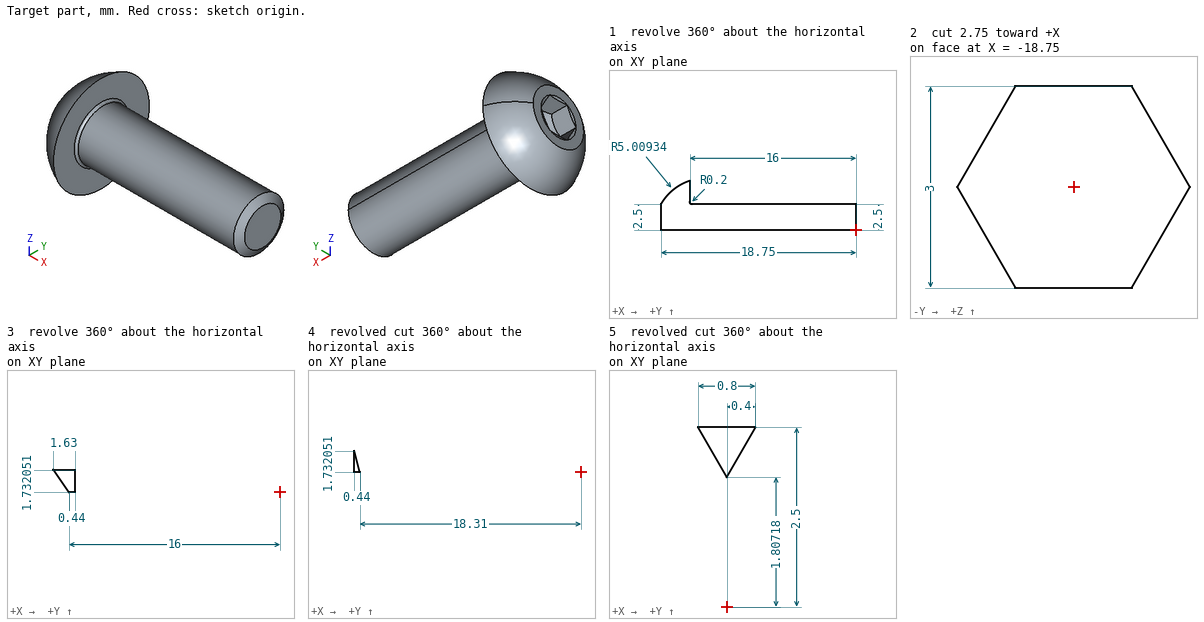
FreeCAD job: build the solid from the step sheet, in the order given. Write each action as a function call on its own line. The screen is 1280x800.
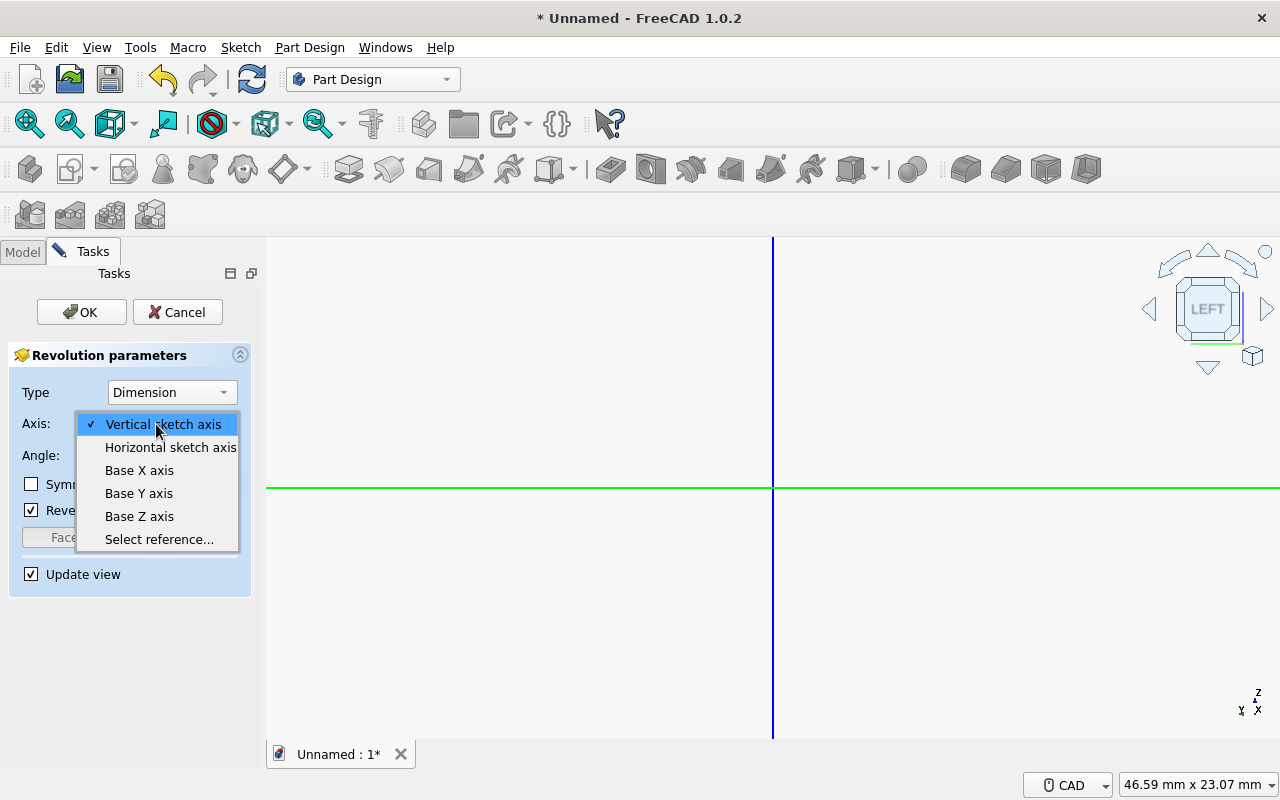
click(156, 448)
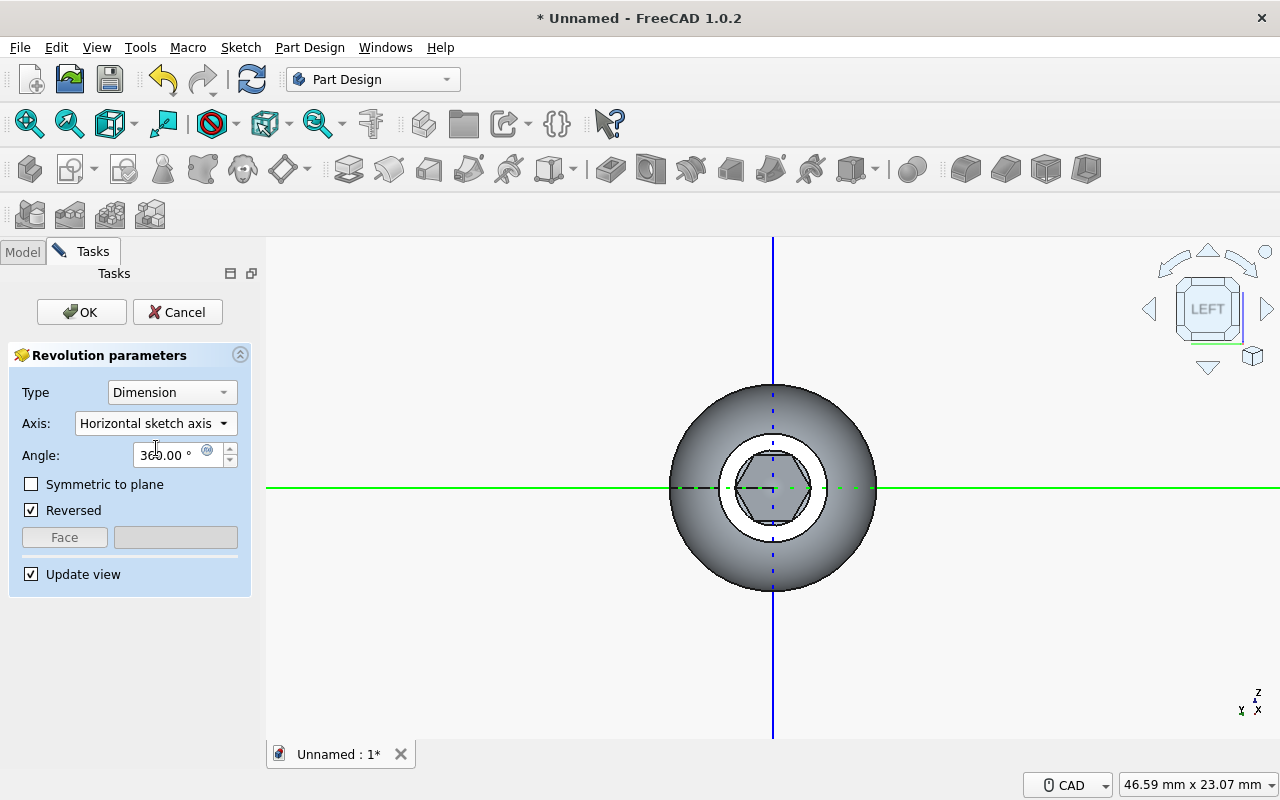
click(82, 312)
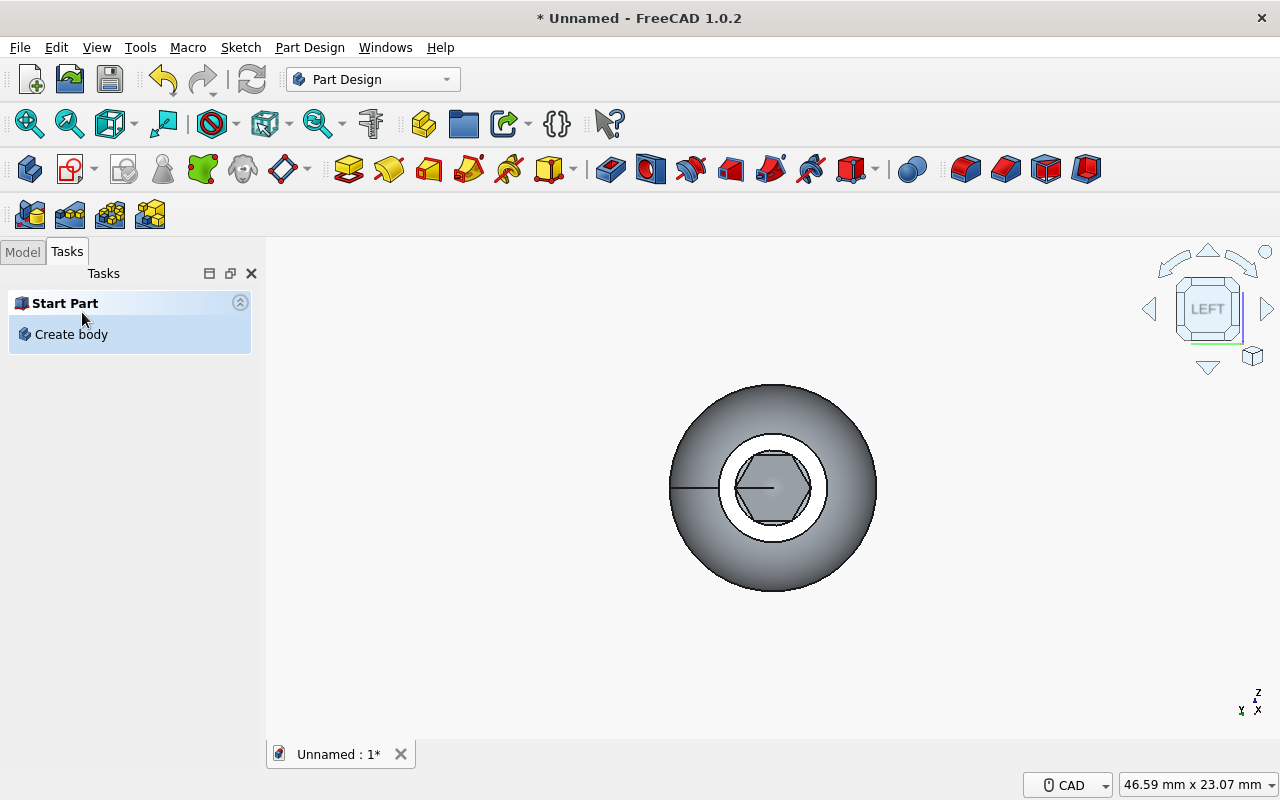
key(0)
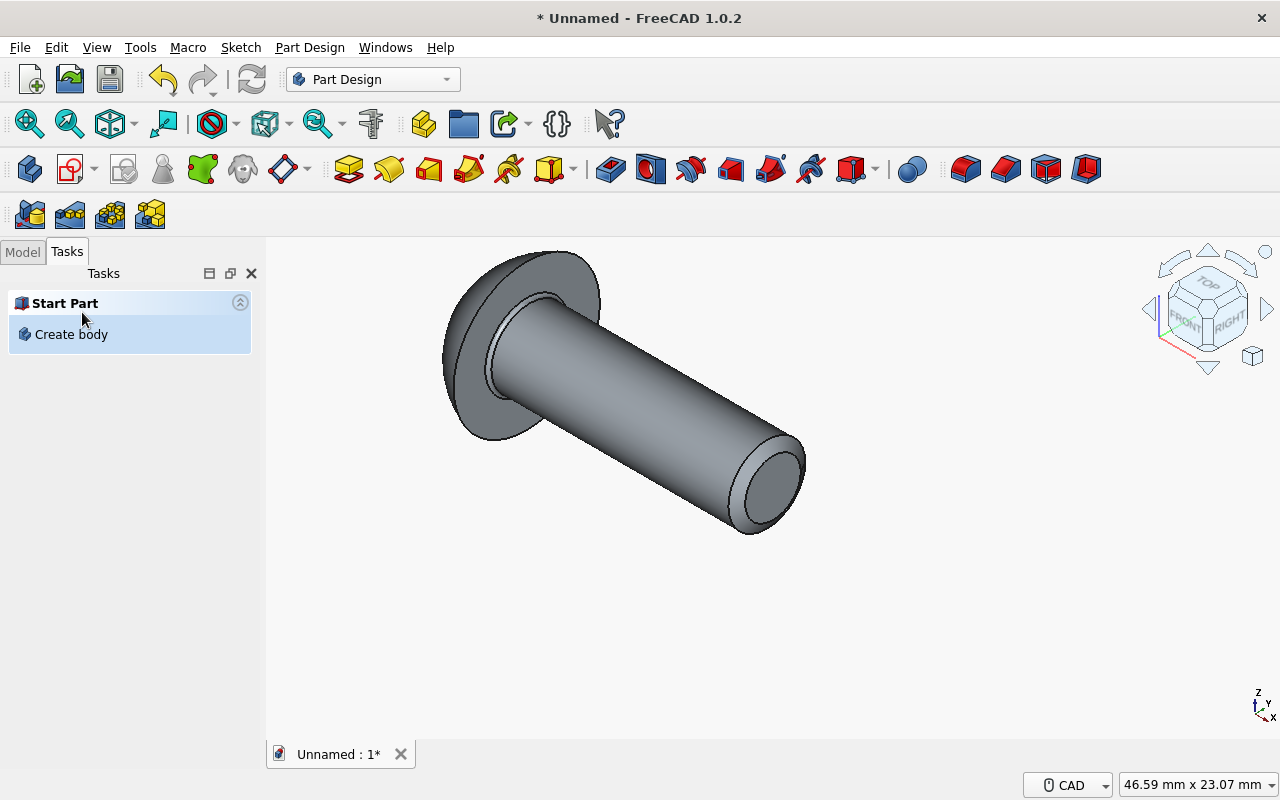
click(30, 124)